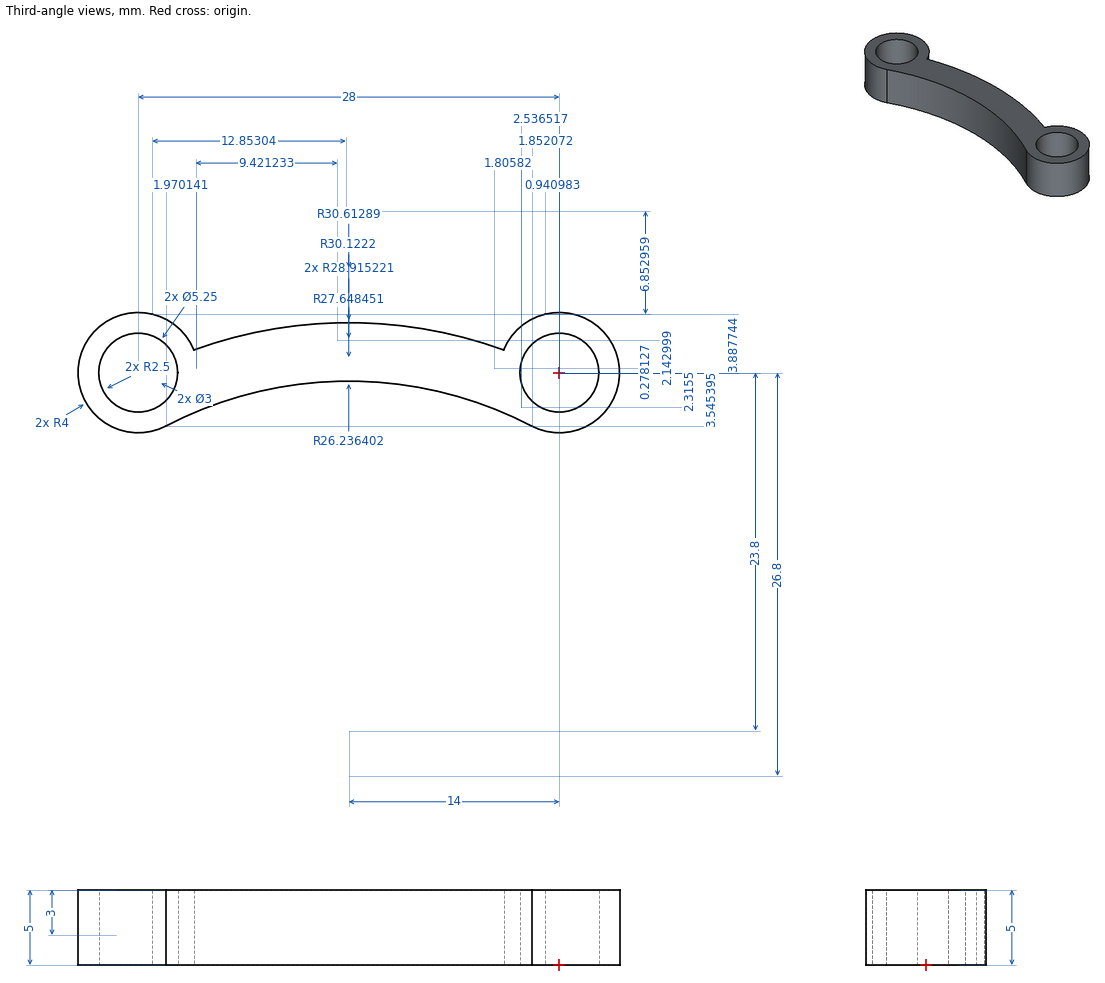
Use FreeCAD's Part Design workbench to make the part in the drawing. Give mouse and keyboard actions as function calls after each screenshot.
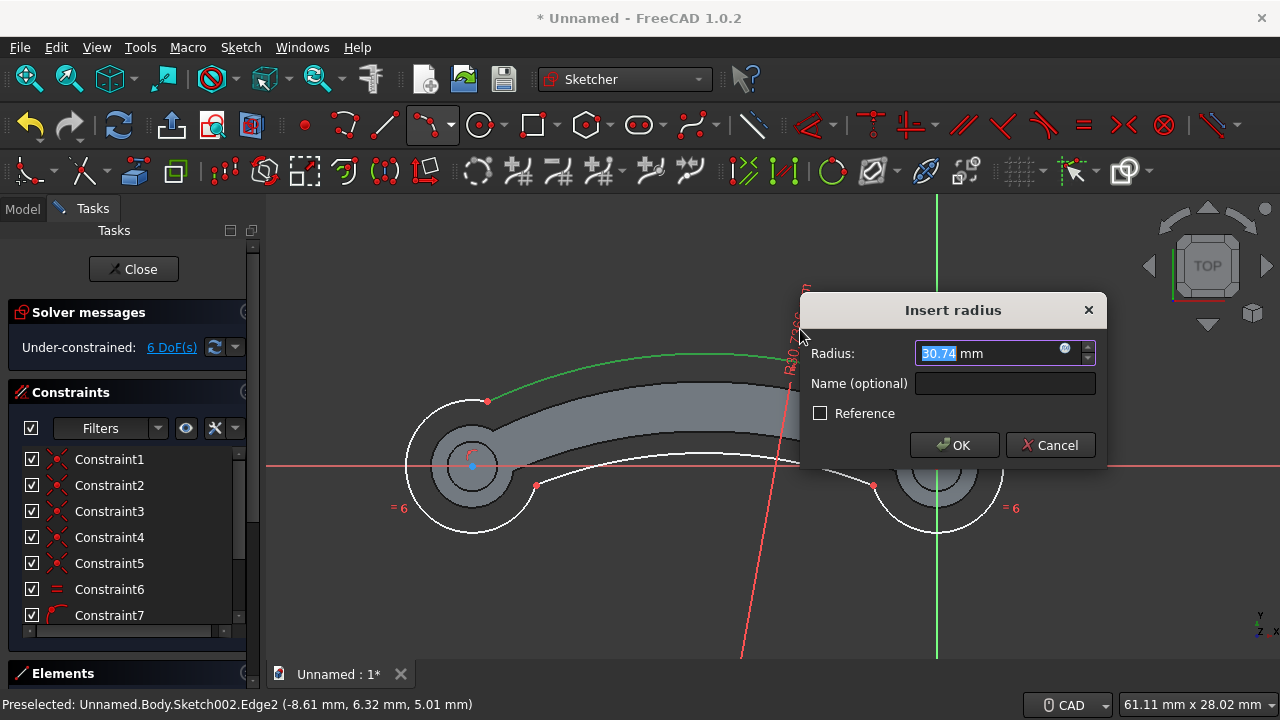
text(30.61289)
key(Return)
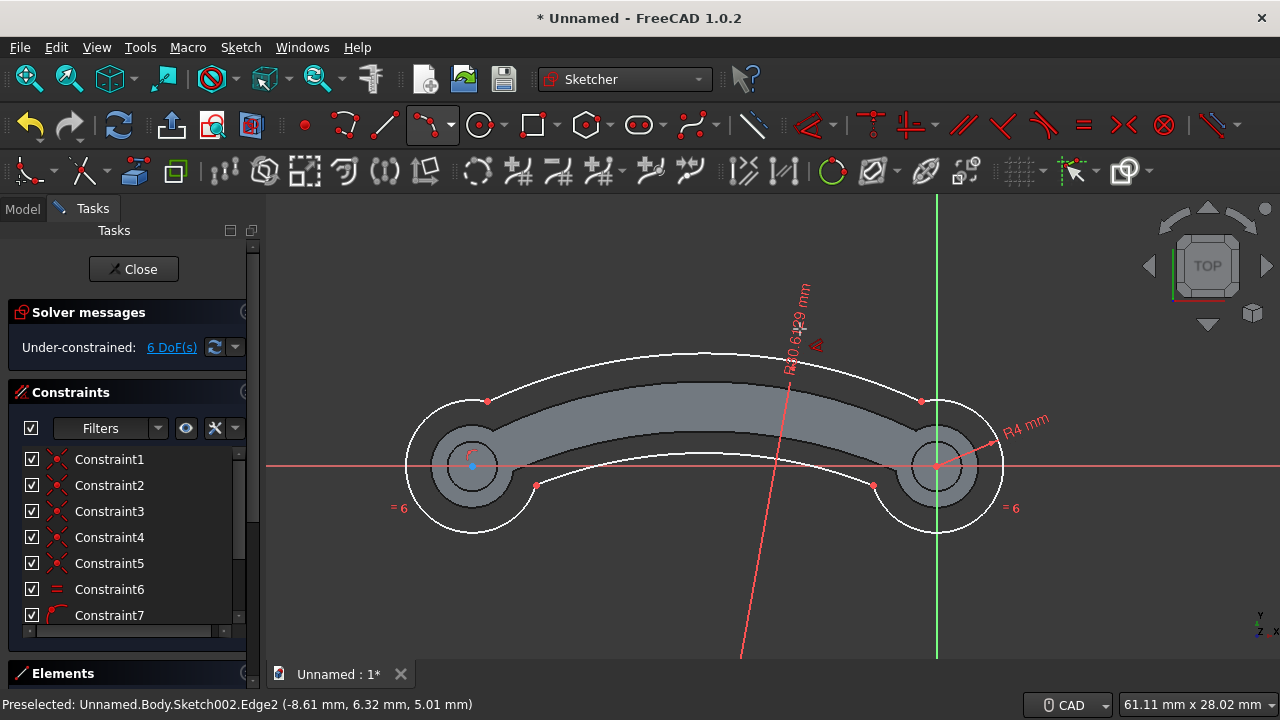
click(705, 453)
click(705, 421)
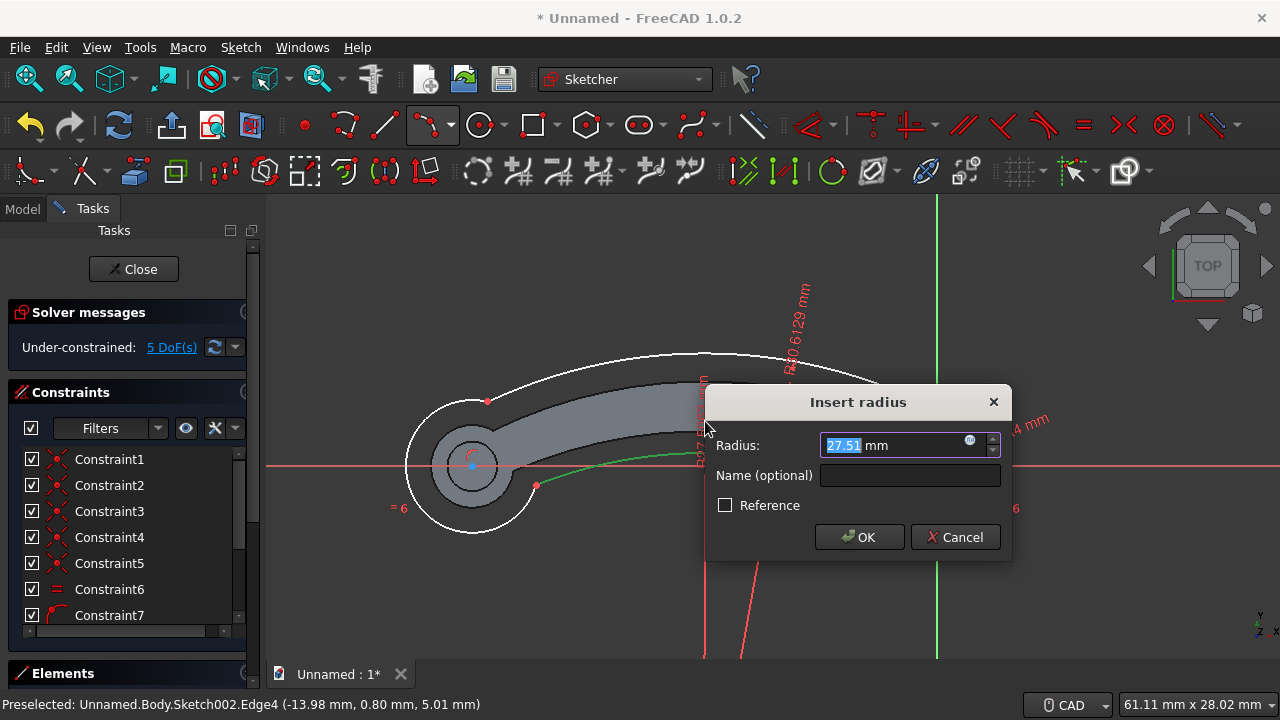
text(27.648451)
key(Return)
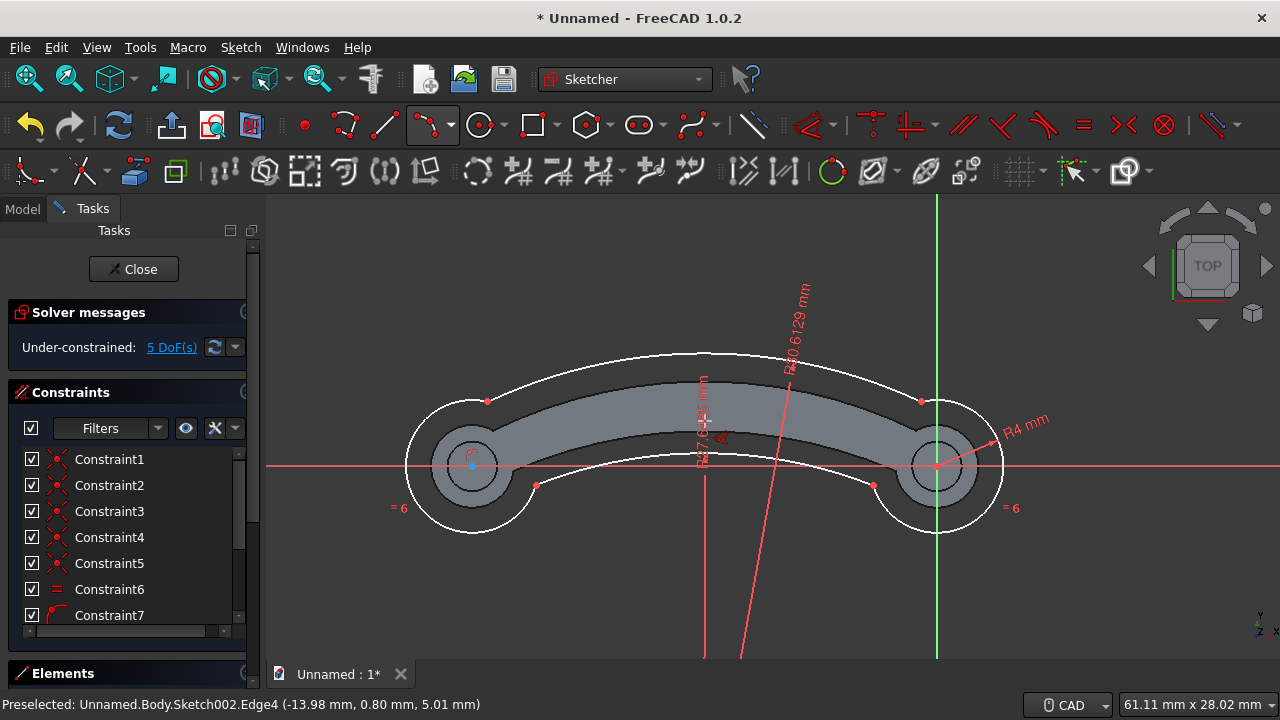
scroll(704, 222, down, 3)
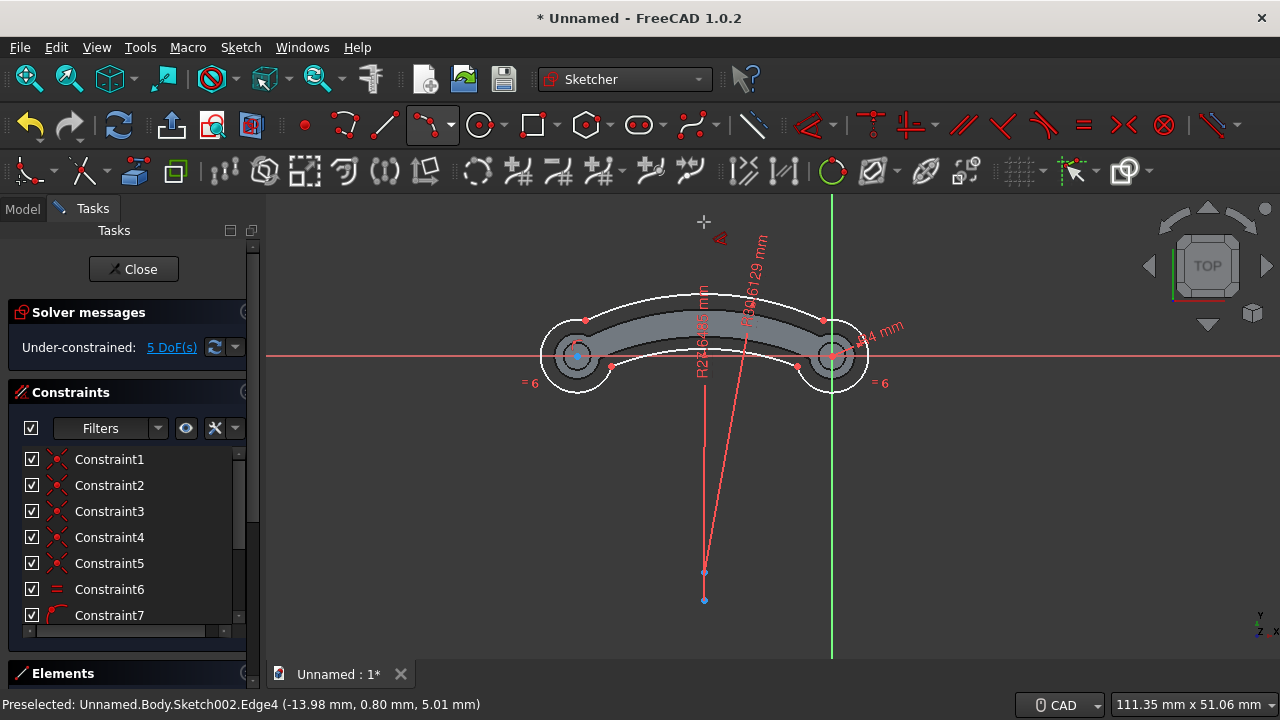
click(704, 573)
click(768, 607)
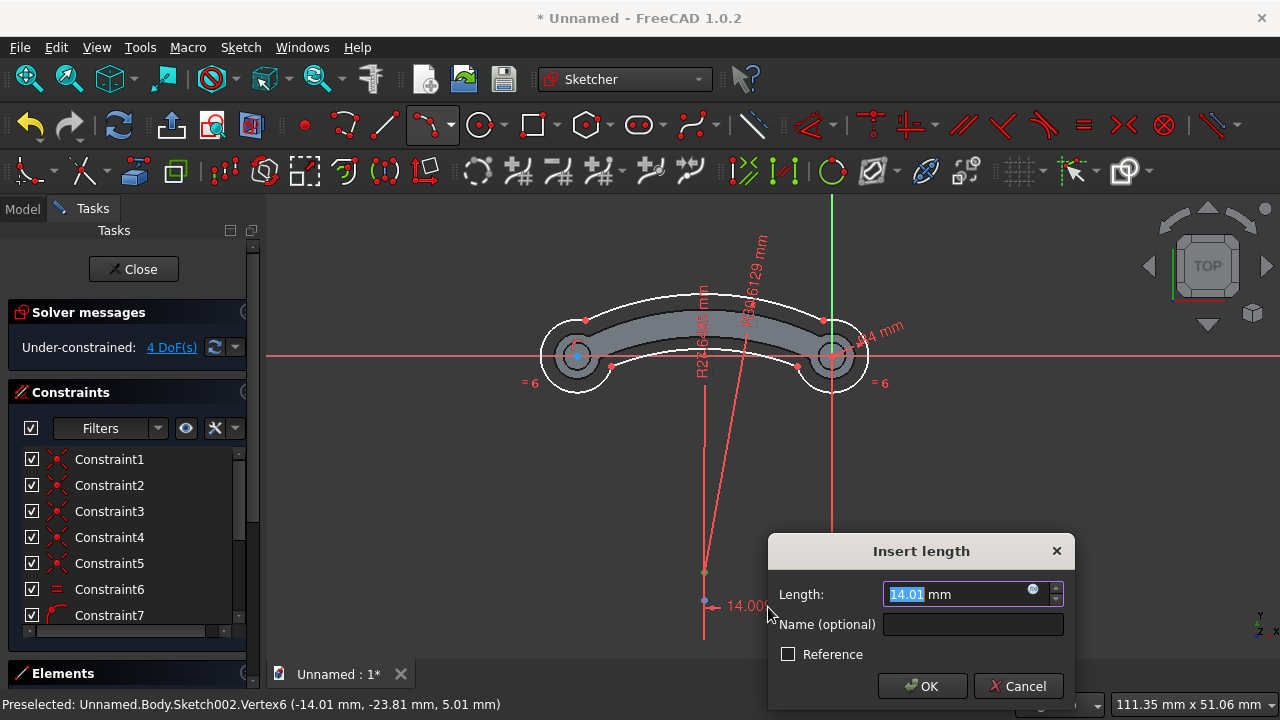
text(14)
key(Return)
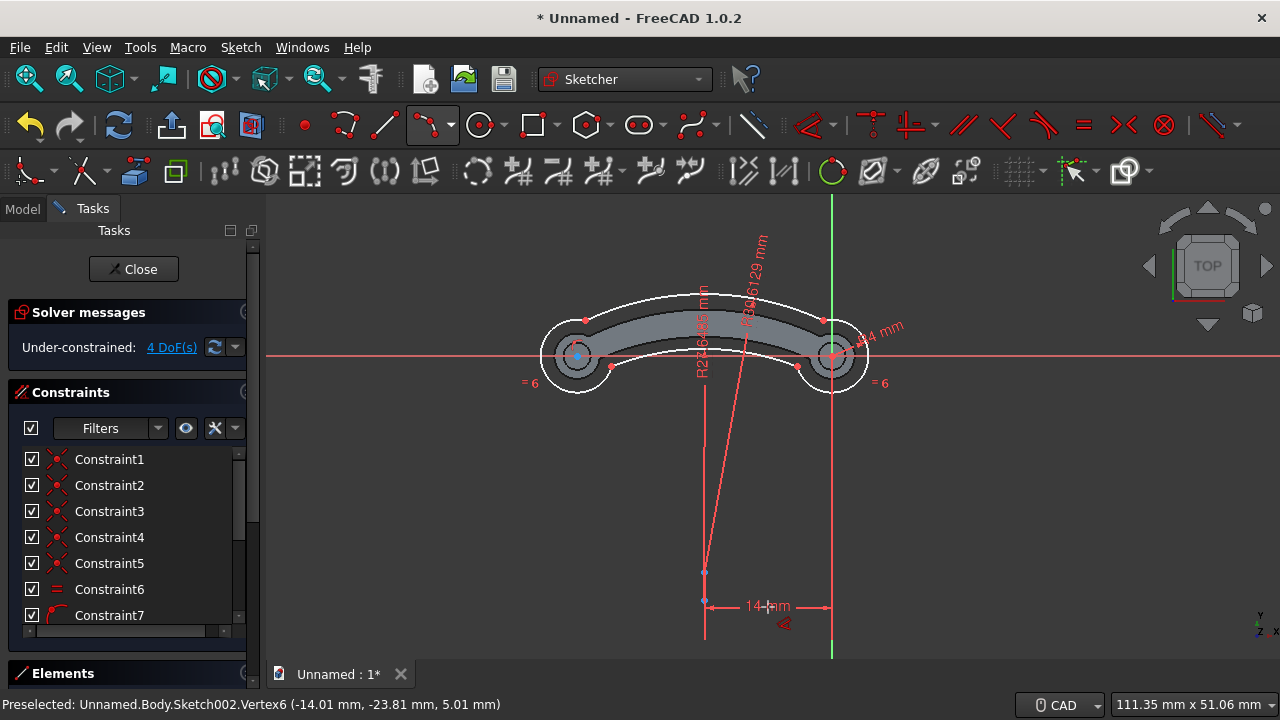
click(577, 356)
click(705, 390)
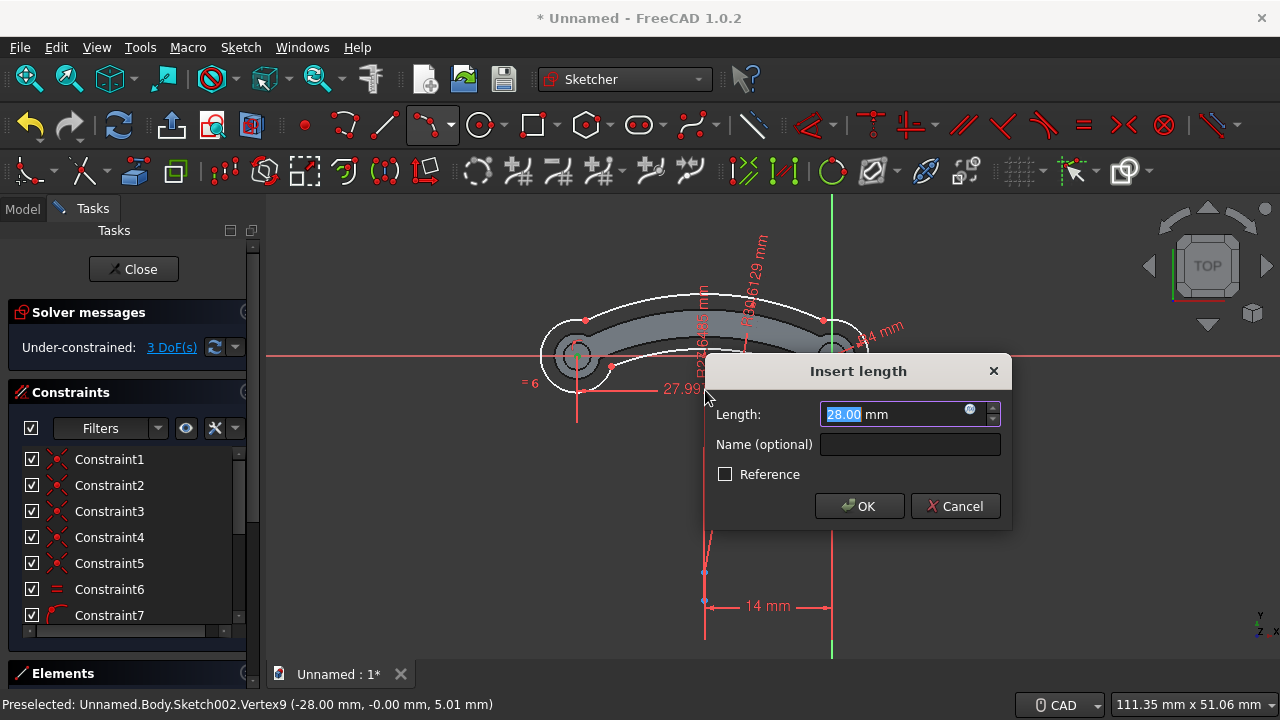
text(28)
key(Return)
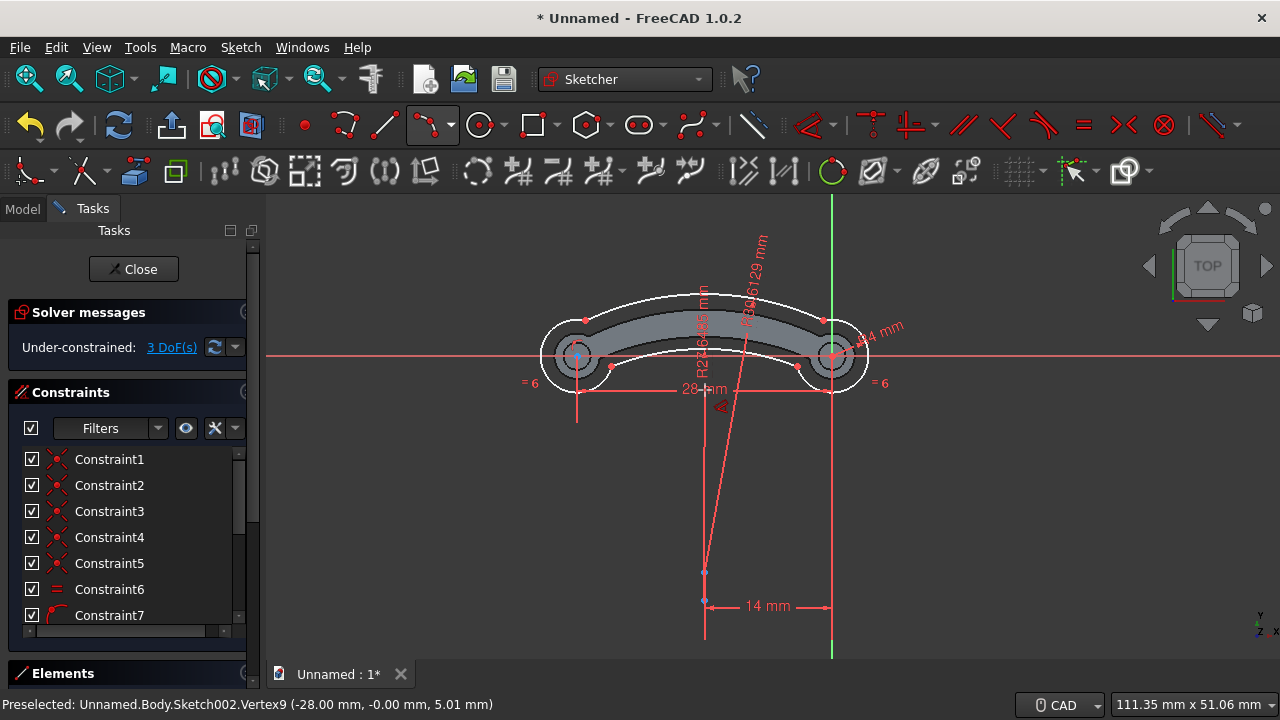
click(704, 601)
click(768, 250)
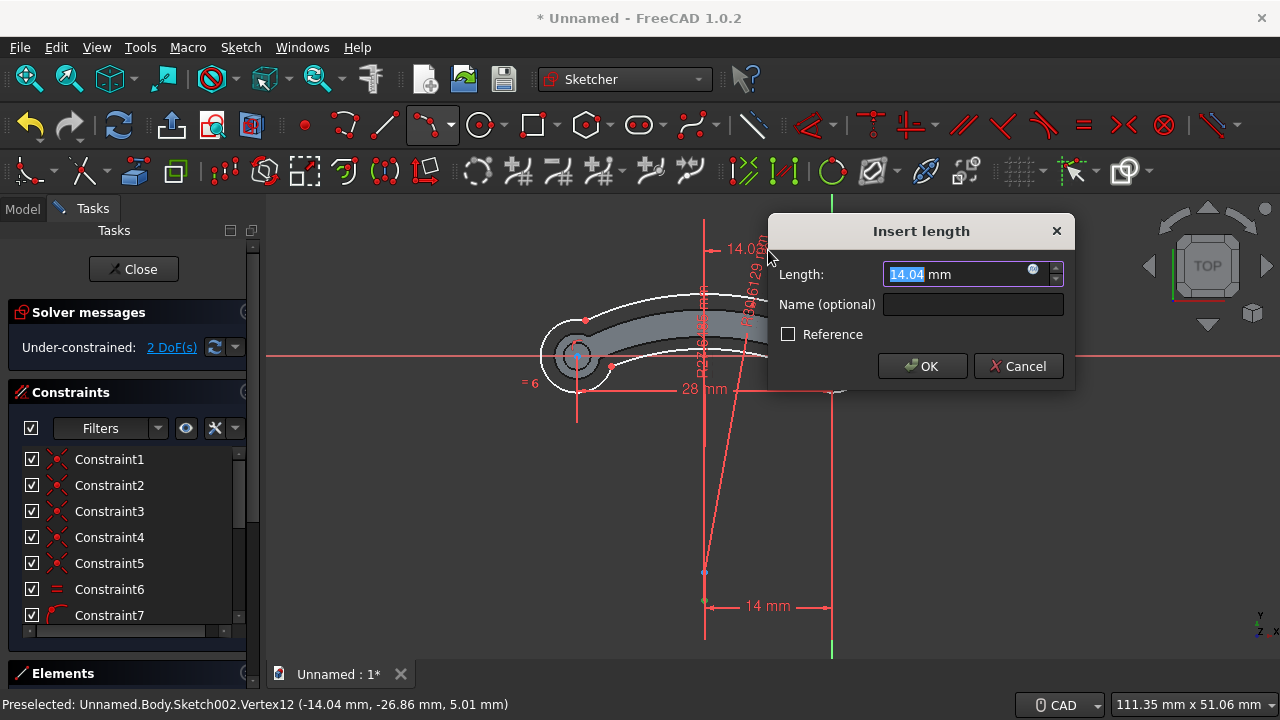
text(14)
key(Return)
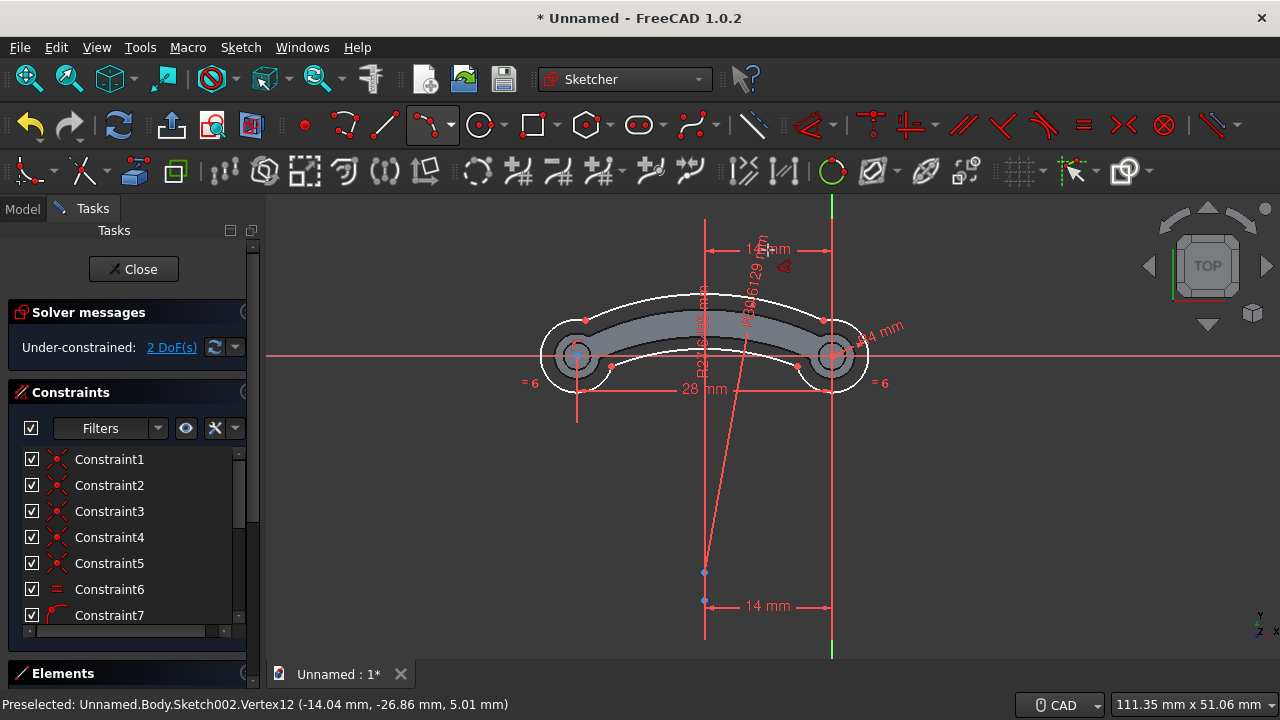
click(705, 573)
click(866, 465)